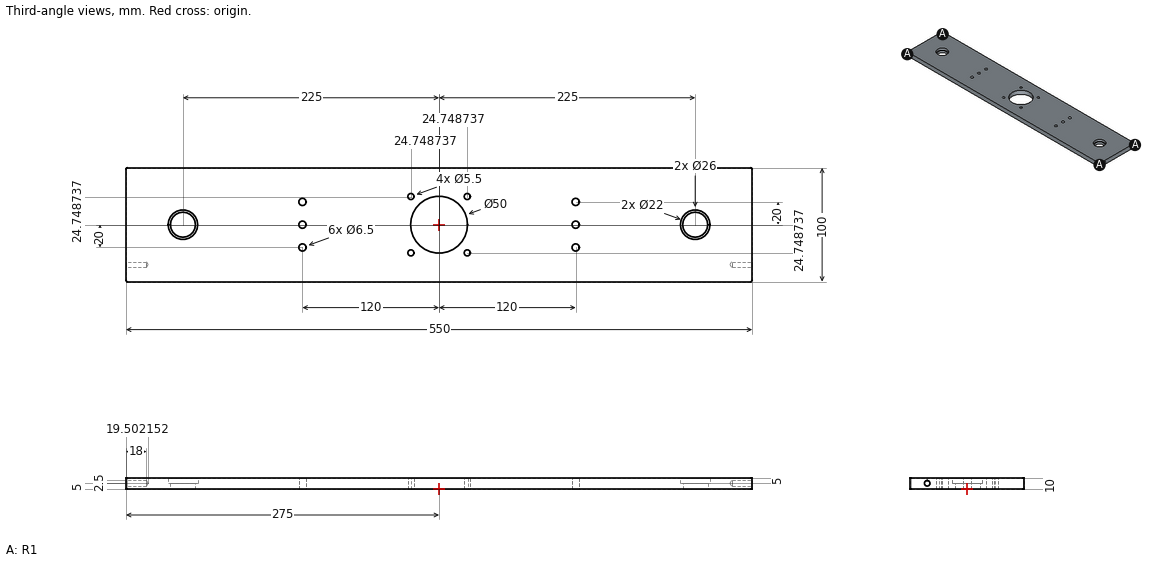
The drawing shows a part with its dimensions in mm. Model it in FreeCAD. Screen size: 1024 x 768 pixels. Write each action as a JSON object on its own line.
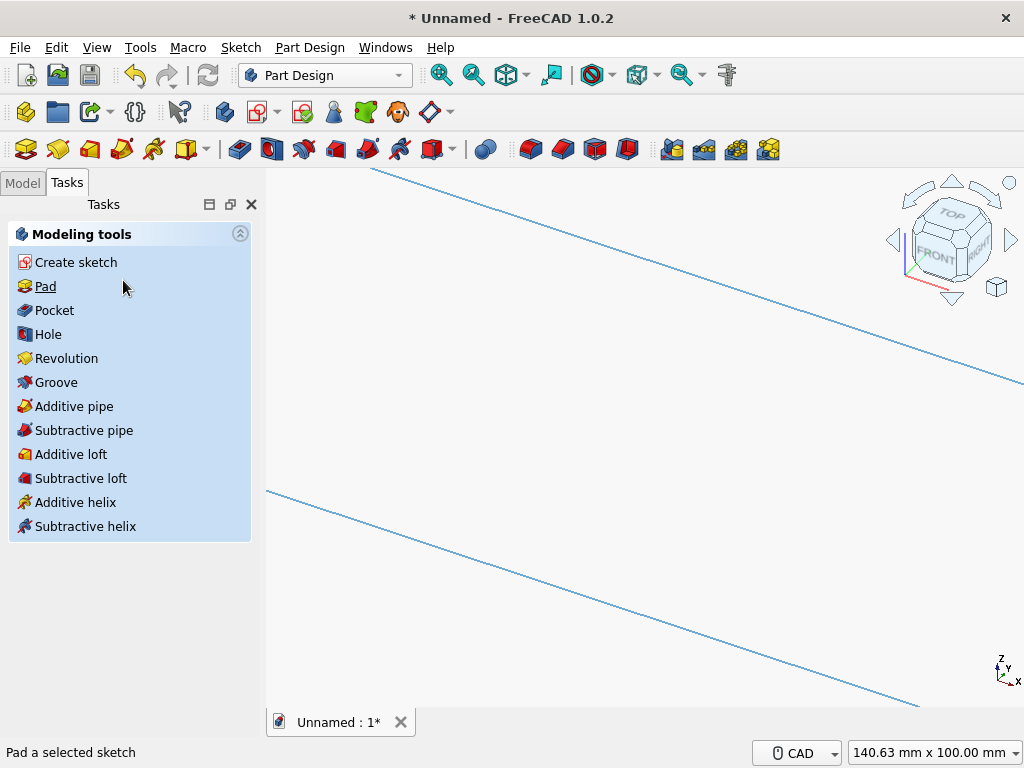
{"action": "left_click", "coordinate": [26, 150]}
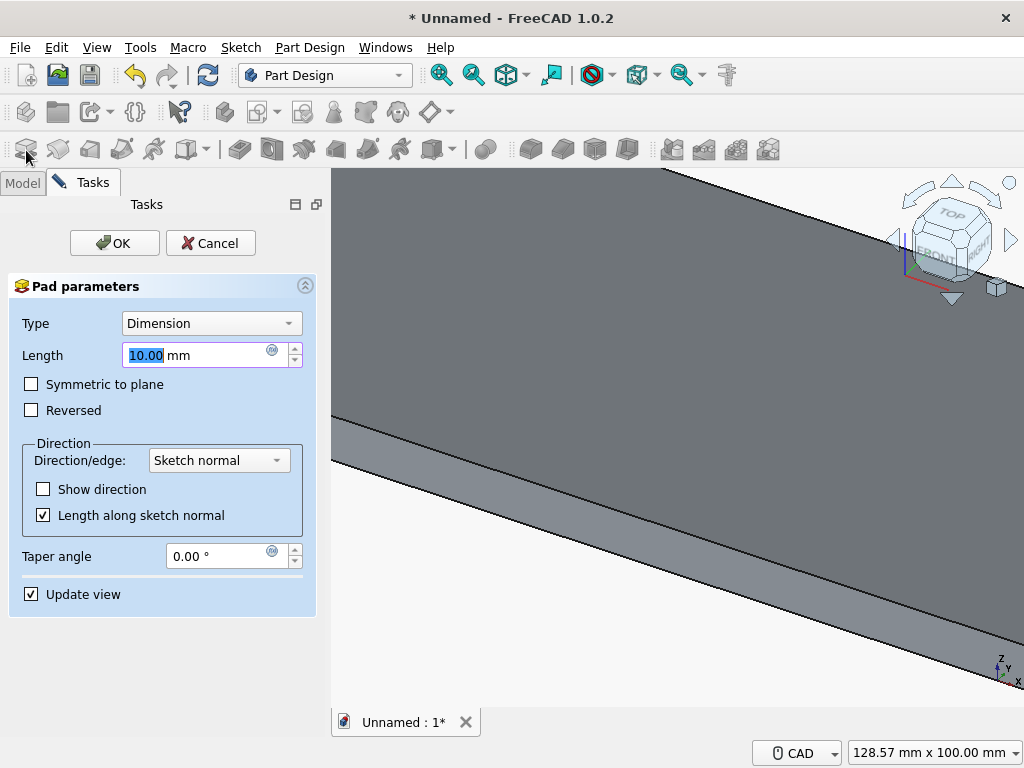
{"action": "type", "text": "10"}
{"action": "key", "text": "Tab"}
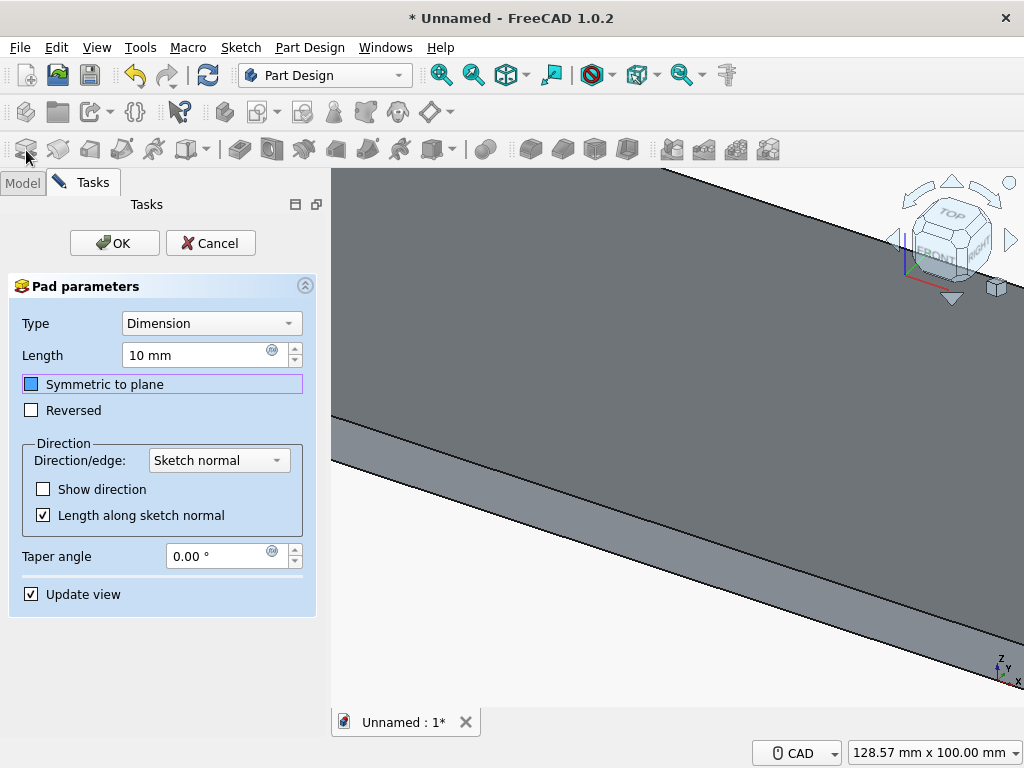
{"action": "left_click", "coordinate": [115, 243]}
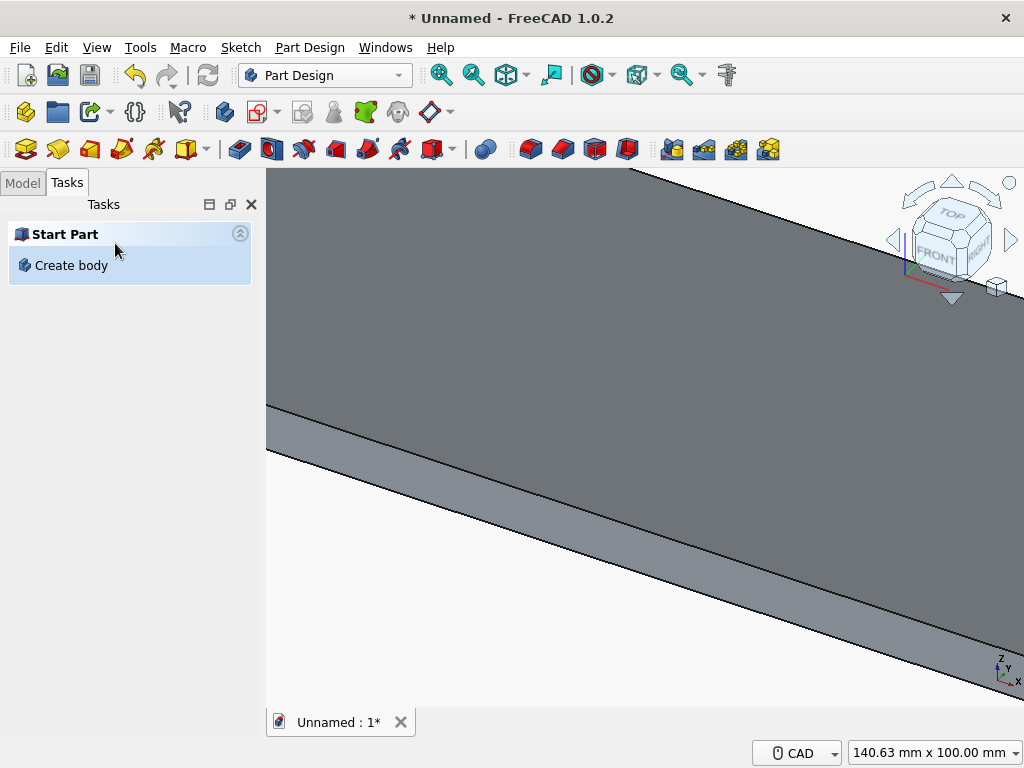
{"action": "left_click", "coordinate": [442, 76]}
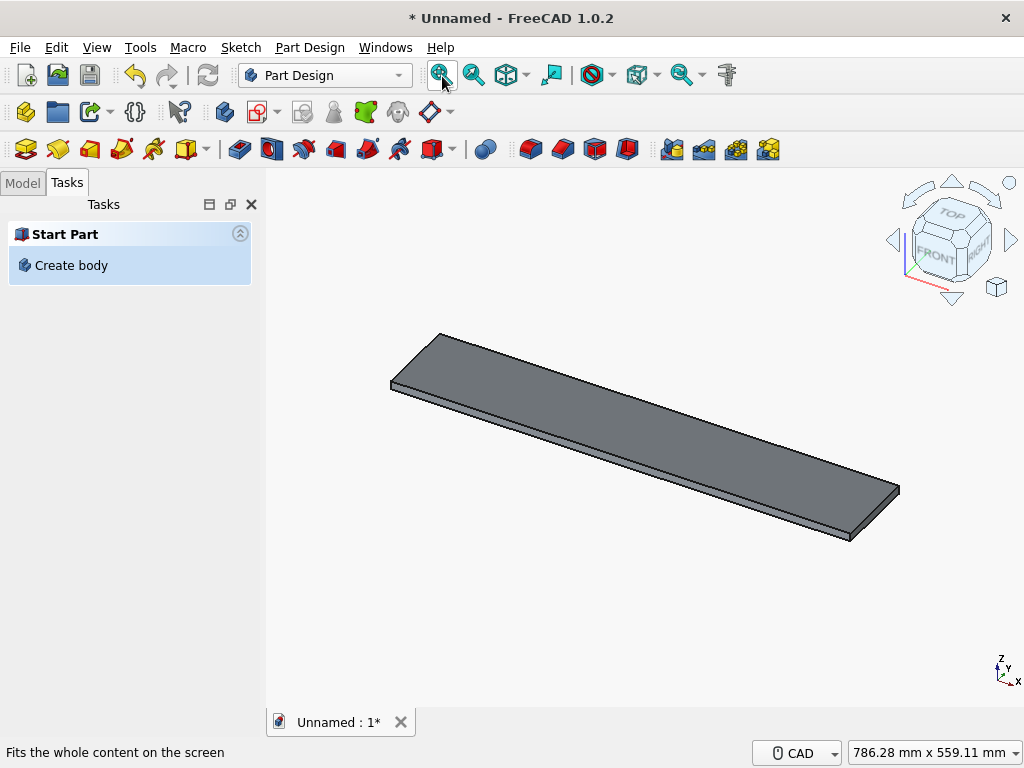
{"action": "left_click", "coordinate": [776, 476]}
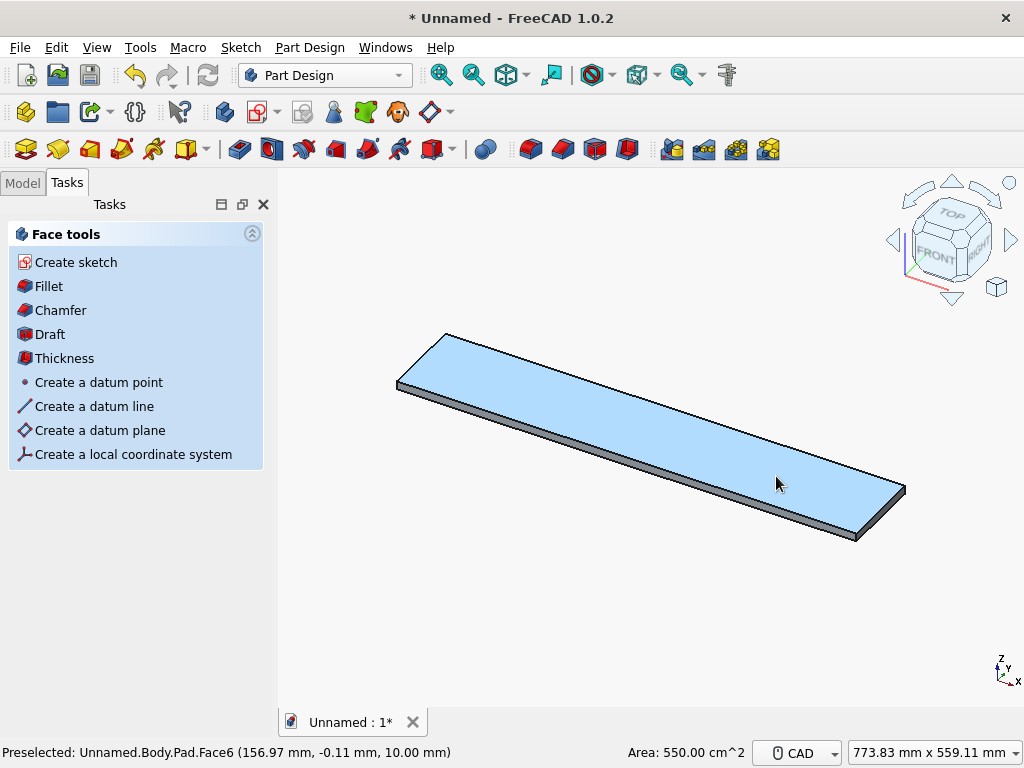
{"action": "left_click", "coordinate": [258, 112]}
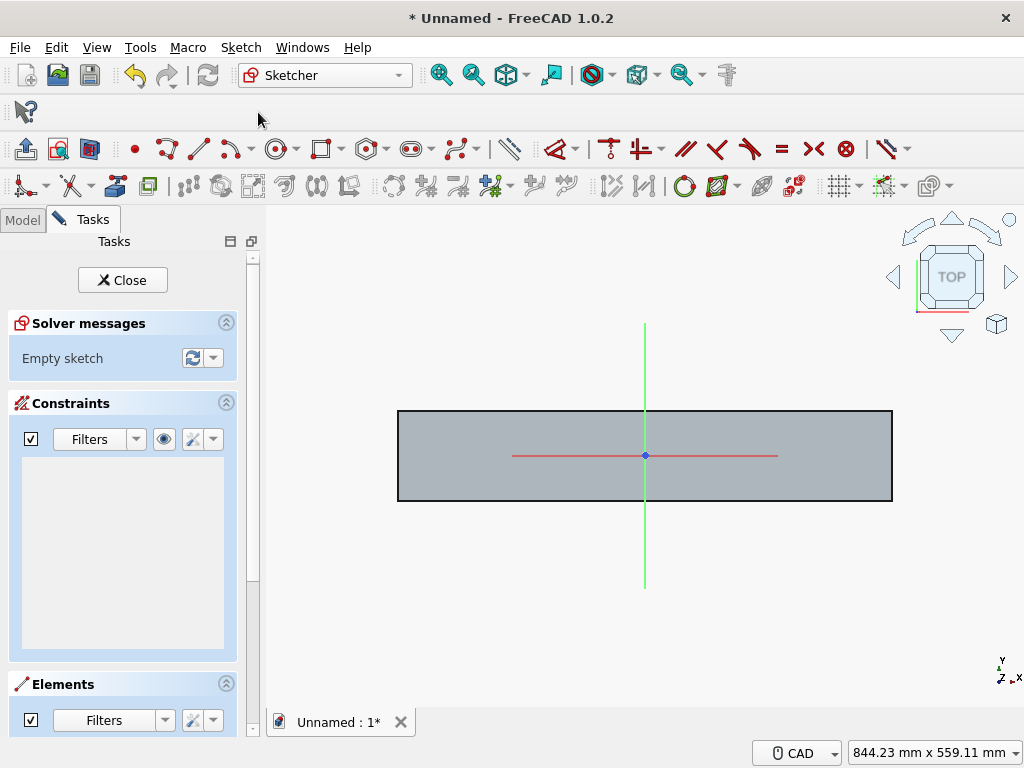
{"action": "scroll", "coordinate": [294, 456], "scroll_direction": "down", "scroll_amount": 1}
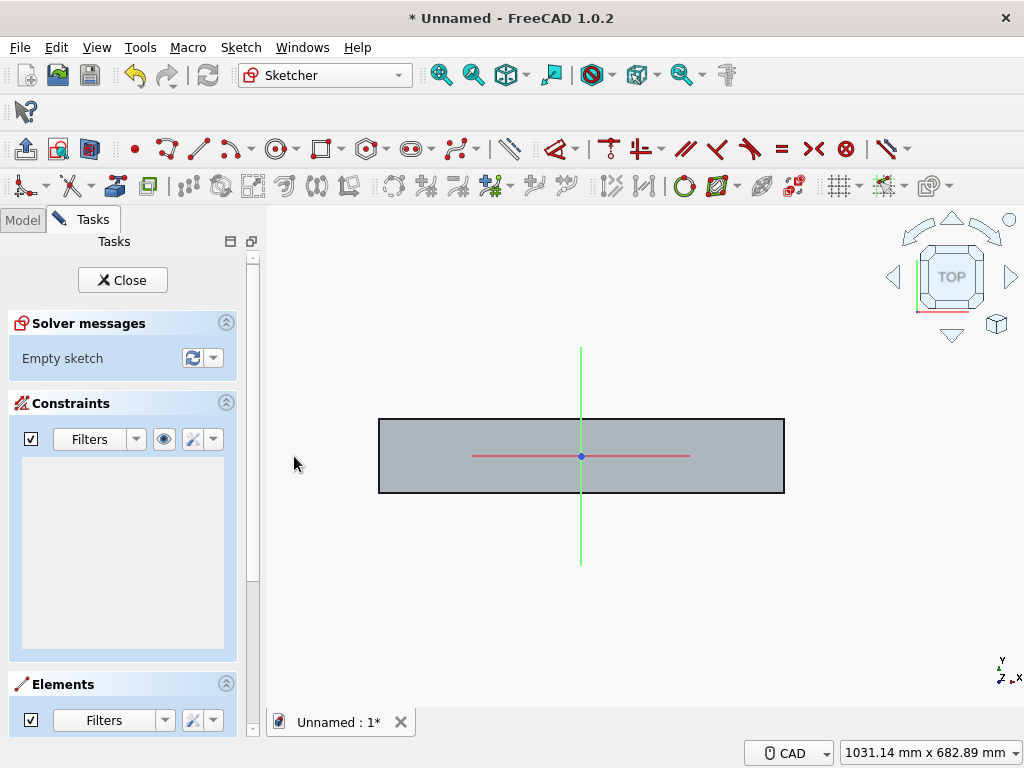
{"action": "left_click", "coordinate": [276, 150]}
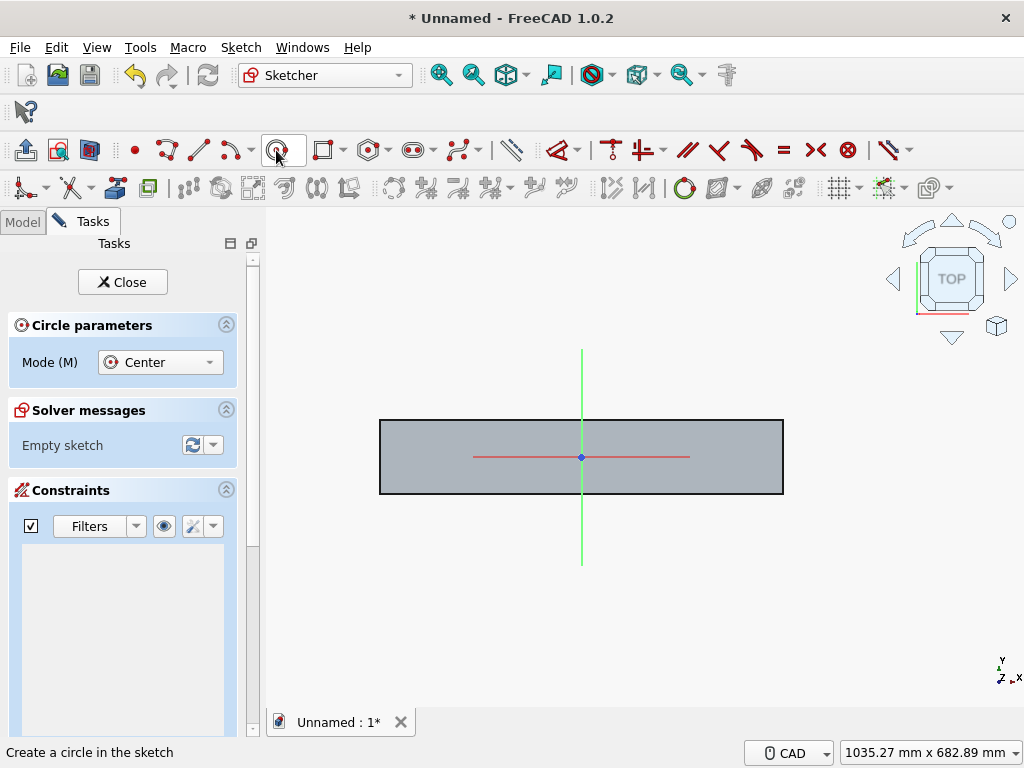
{"action": "scroll", "coordinate": [746, 457], "scroll_direction": "up", "scroll_amount": 5}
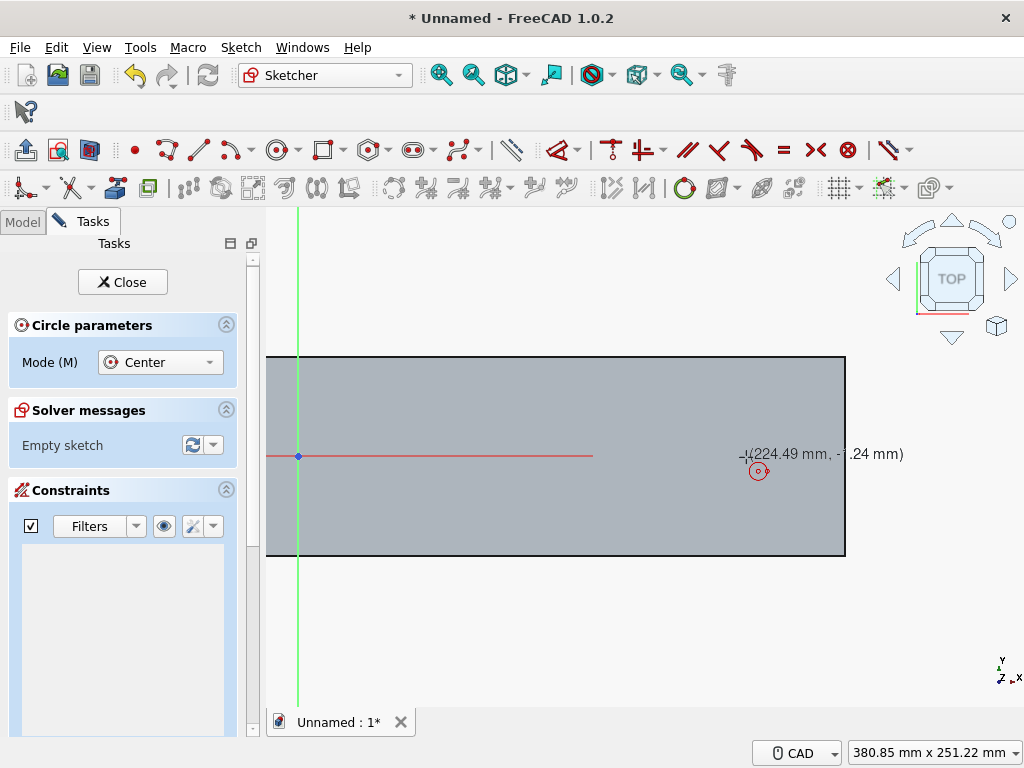
{"action": "left_click", "coordinate": [746, 456]}
{"action": "left_click", "coordinate": [764, 438]}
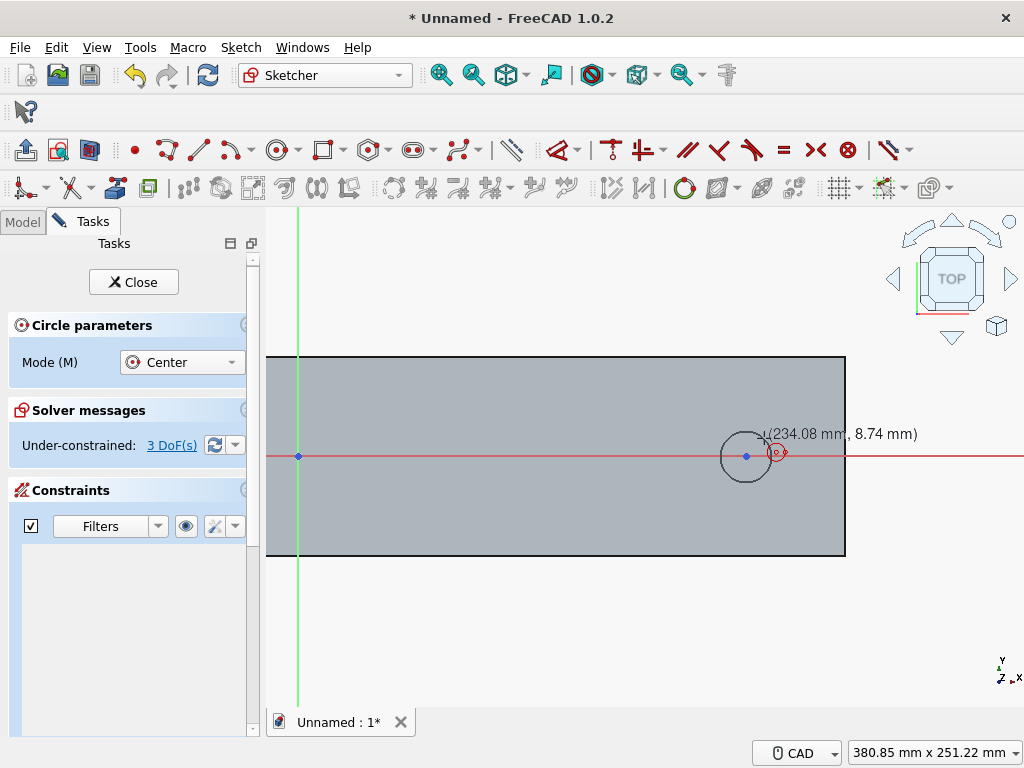
{"action": "scroll", "coordinate": [804, 458], "scroll_direction": "down", "scroll_amount": 4}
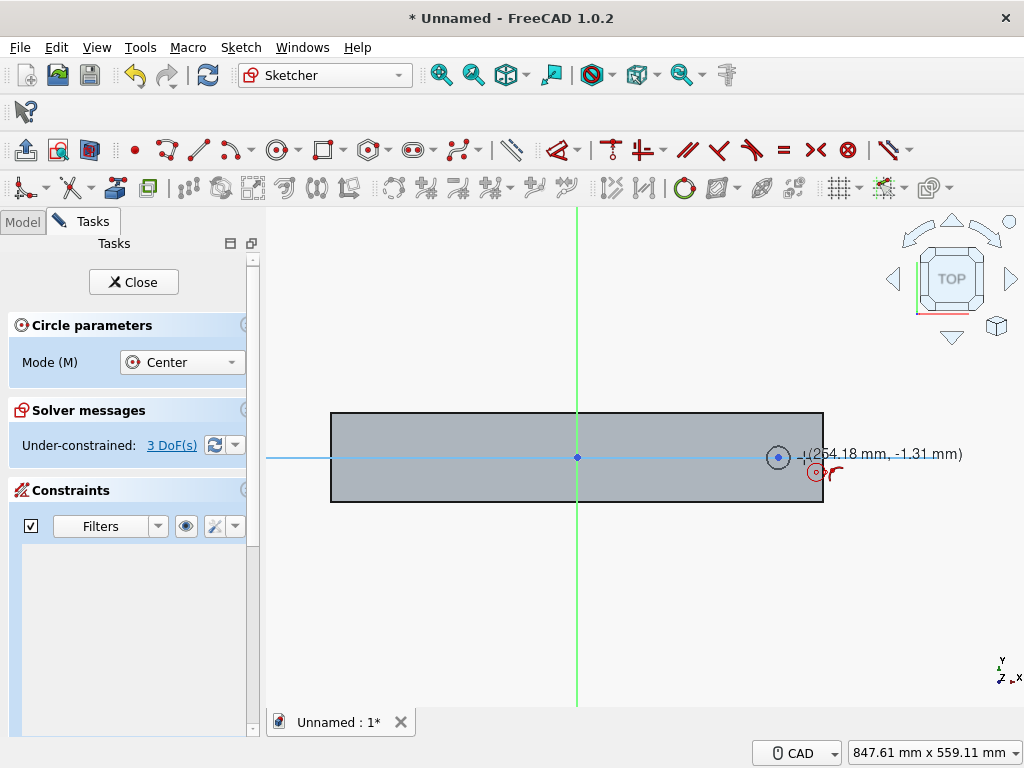
{"action": "scroll", "coordinate": [376, 458], "scroll_direction": "up", "scroll_amount": 4}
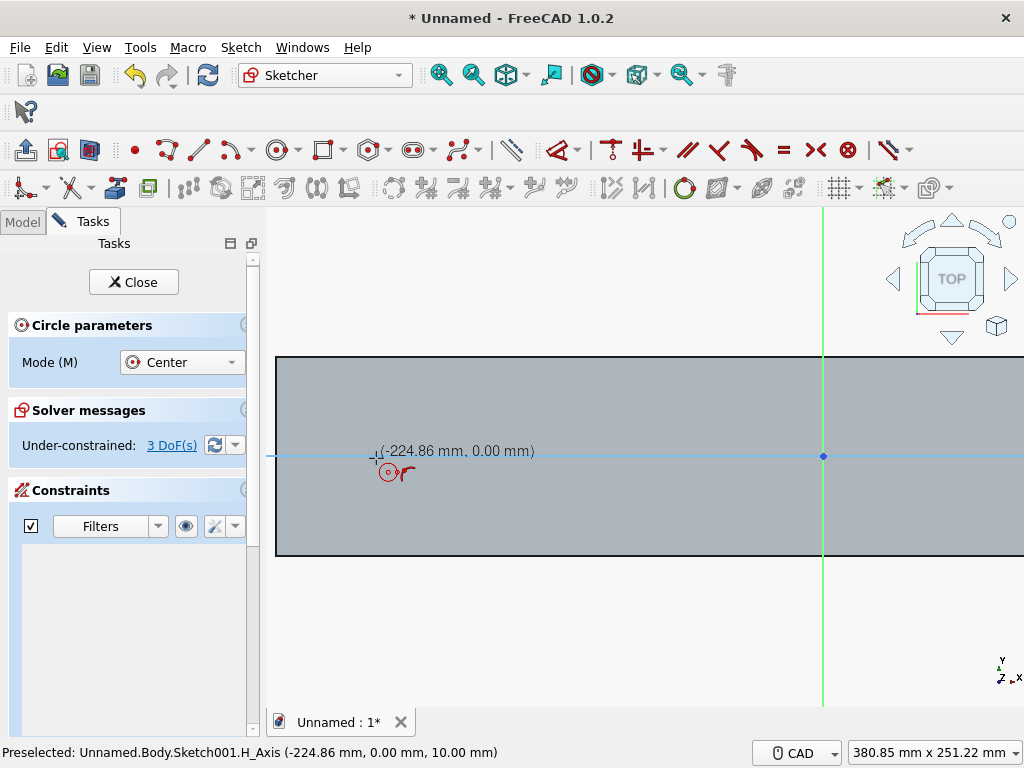
{"action": "left_click", "coordinate": [376, 456]}
{"action": "left_click", "coordinate": [394, 438]}
{"action": "key", "text": "Escape"}